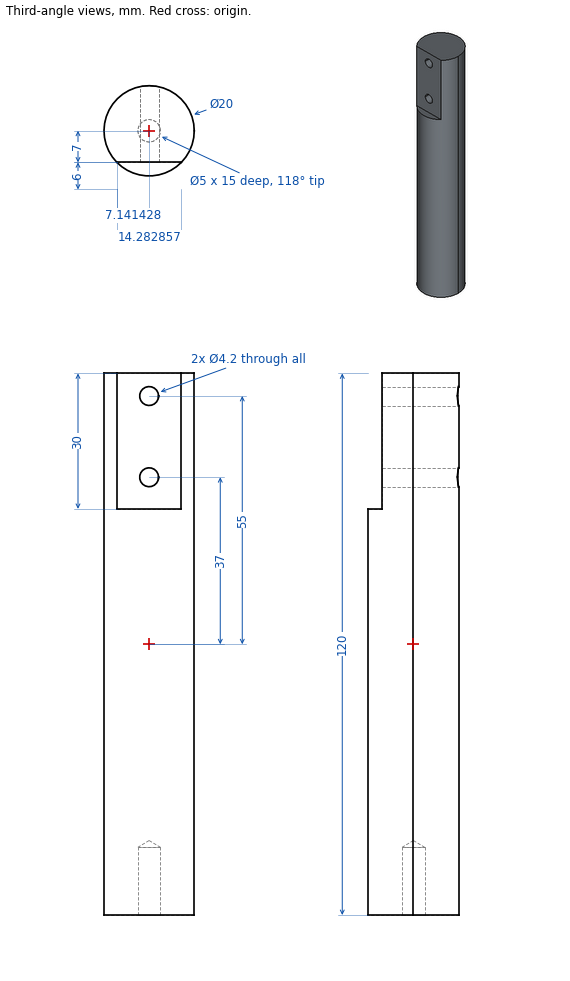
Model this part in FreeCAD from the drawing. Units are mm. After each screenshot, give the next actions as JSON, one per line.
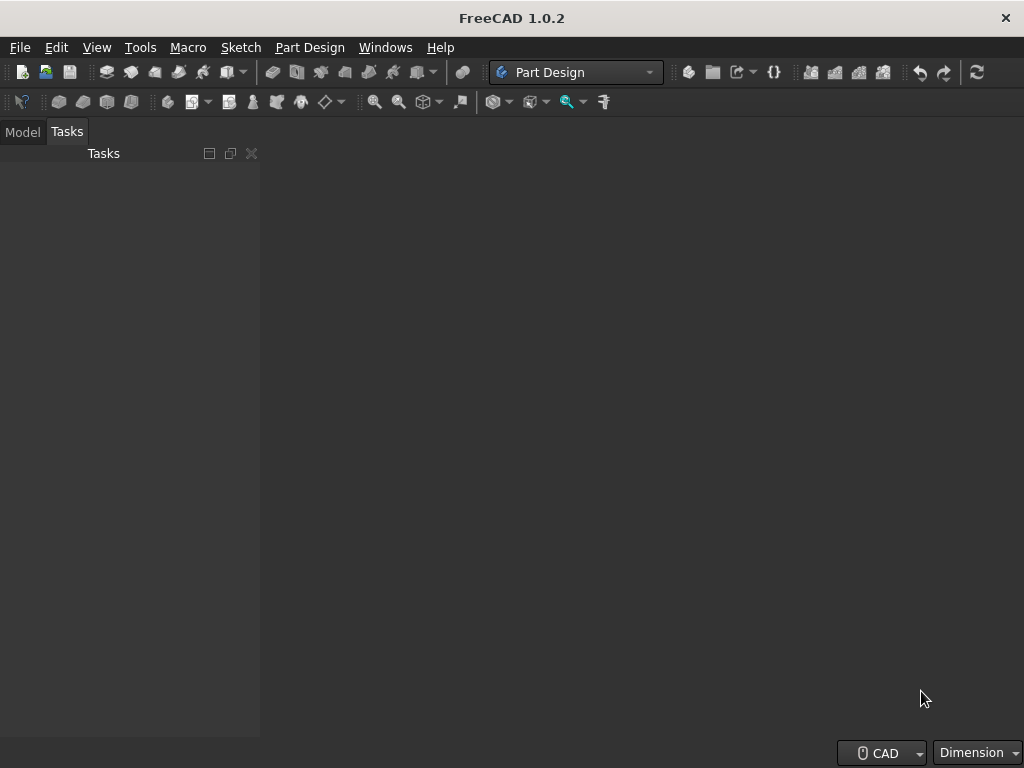
{"action": "left_click", "coordinate": [22, 72]}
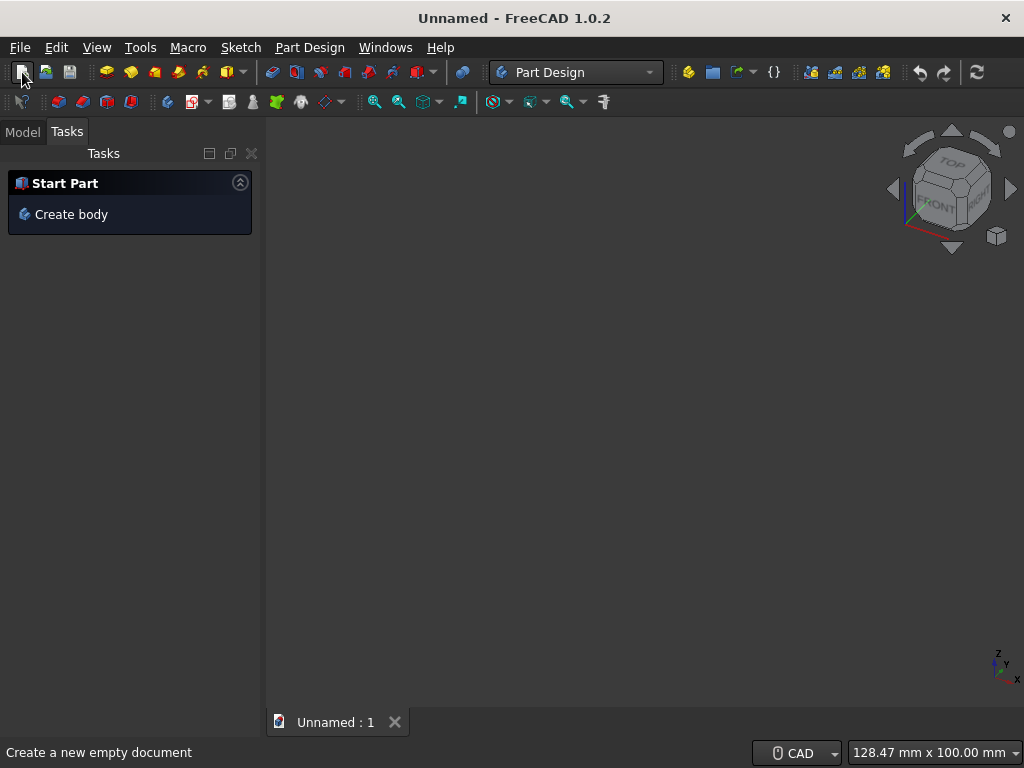
{"action": "left_click", "coordinate": [192, 102]}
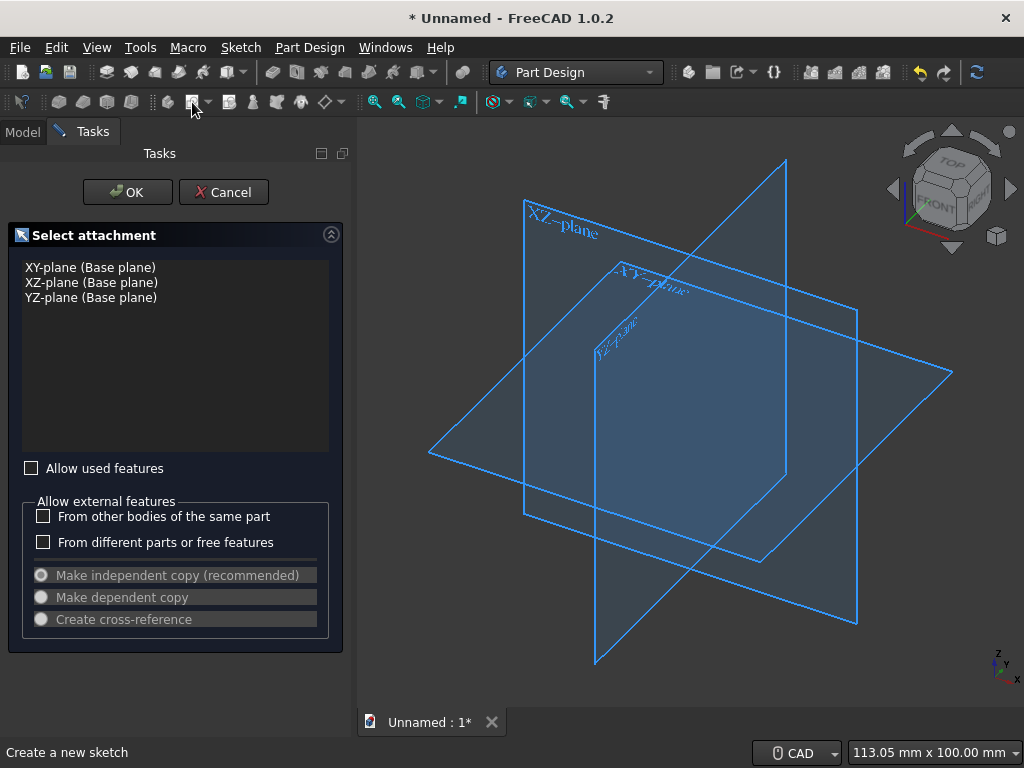
{"action": "left_click", "coordinate": [82, 268]}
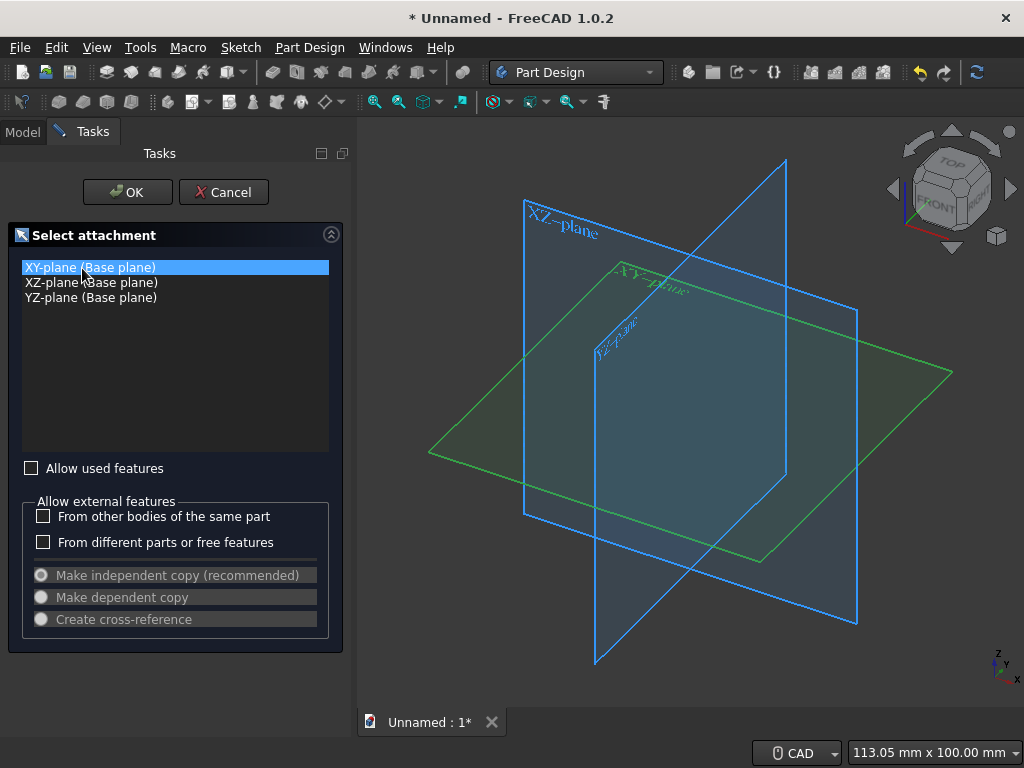
{"action": "left_click", "coordinate": [128, 192]}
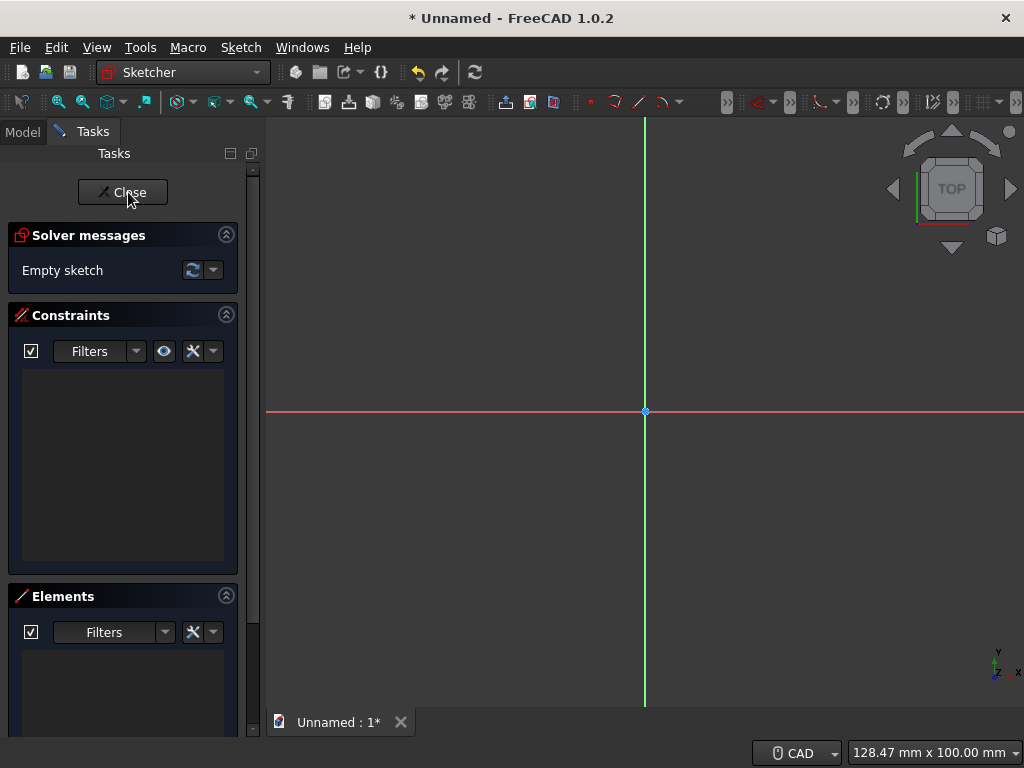
{"action": "scroll", "coordinate": [675, 412], "scroll_direction": "up", "scroll_amount": 6}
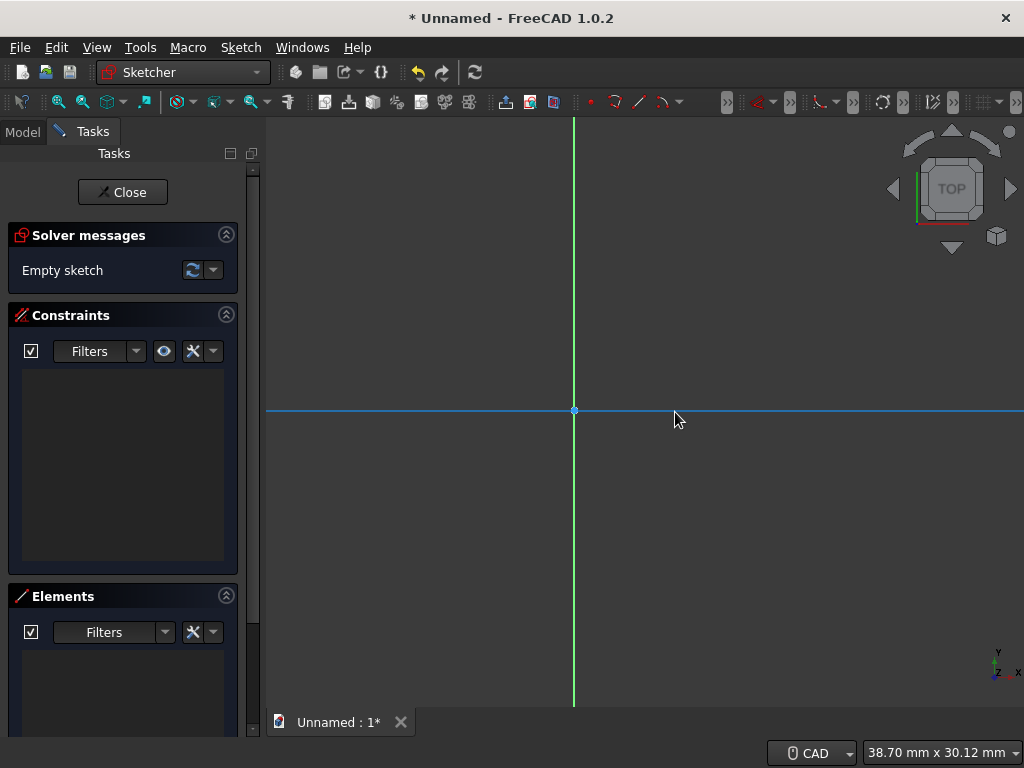
{"action": "key", "text": "g c"}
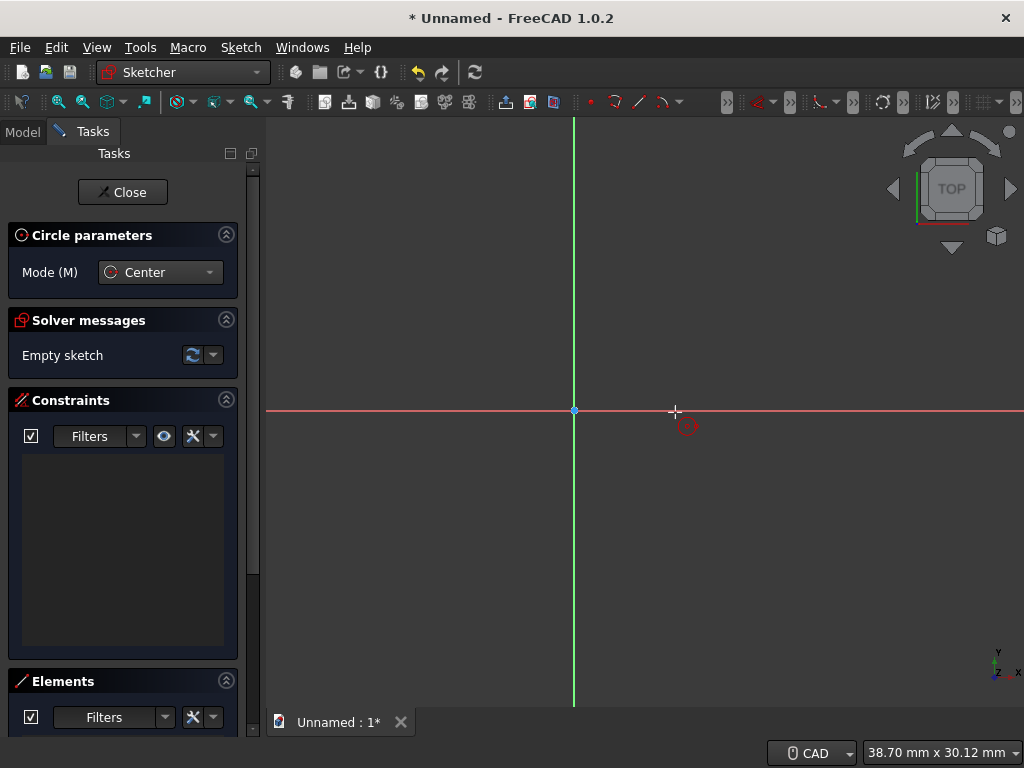
{"action": "left_click", "coordinate": [574, 411]}
{"action": "left_click", "coordinate": [713, 272]}
{"action": "key", "text": "Escape"}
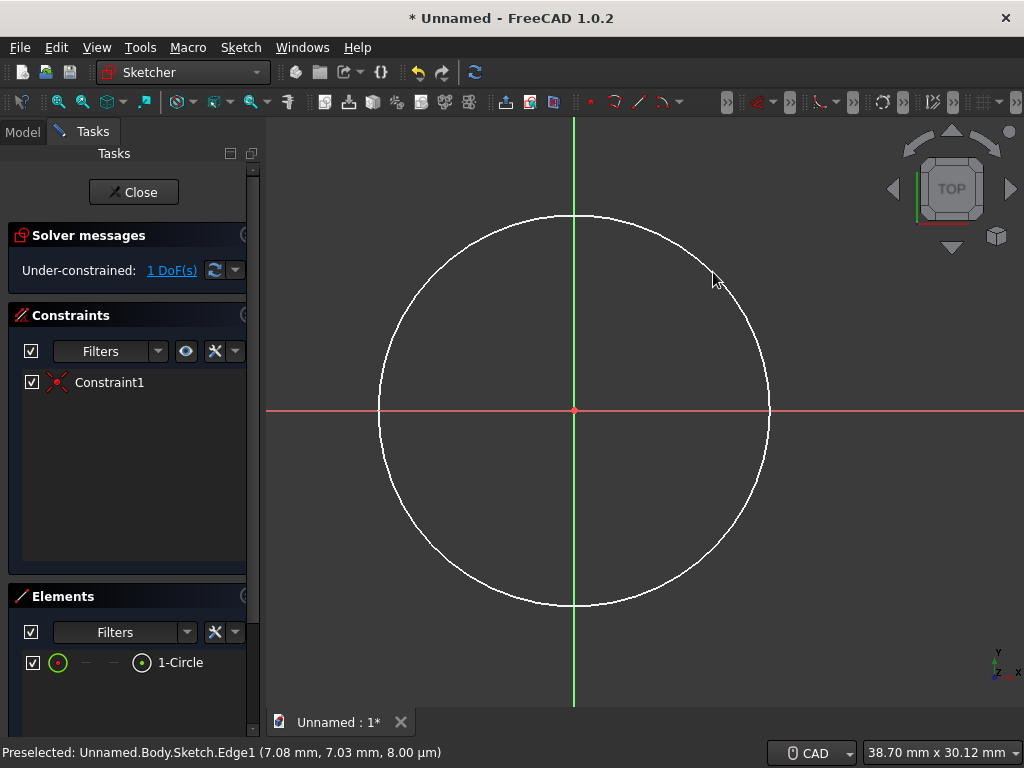
{"action": "left_click", "coordinate": [758, 102]}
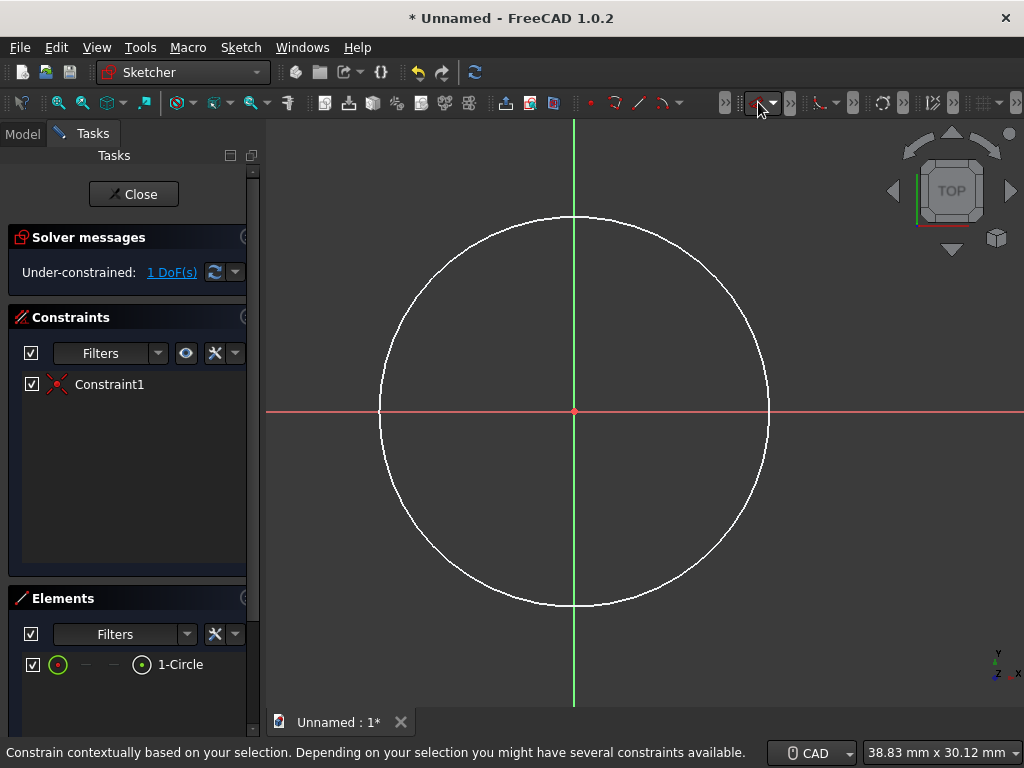
{"action": "left_click", "coordinate": [712, 274]}
{"action": "left_click", "coordinate": [735, 251]}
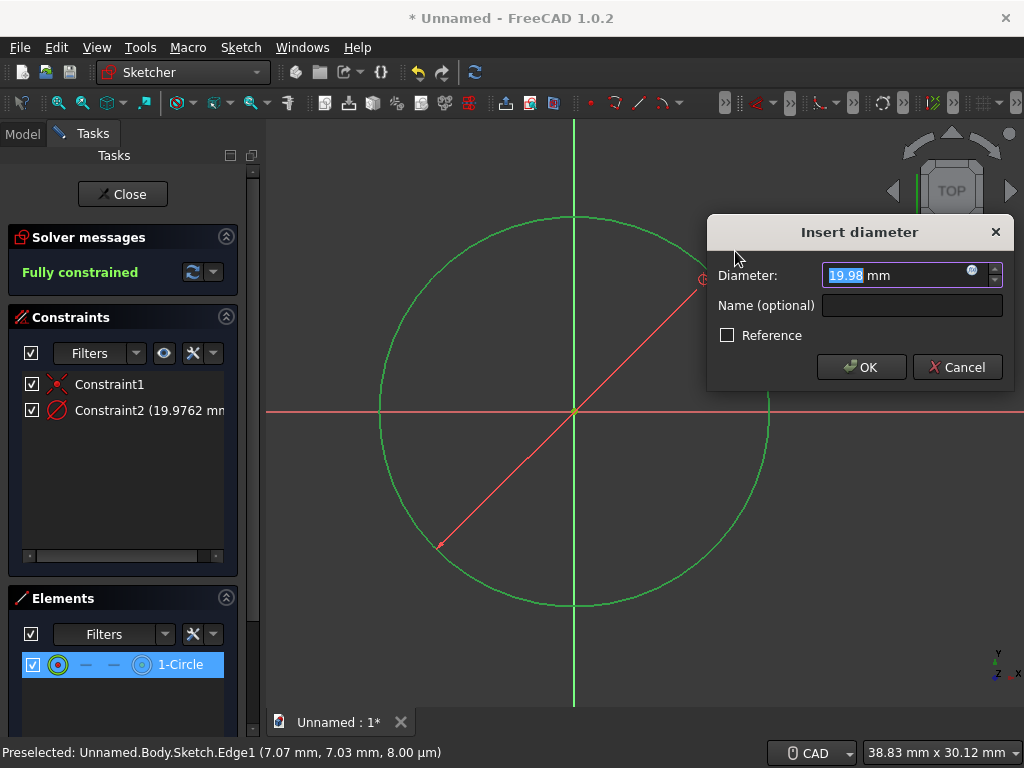
{"action": "type", "text": "20"}
{"action": "key", "text": "Return"}
{"action": "key", "text": "Escape"}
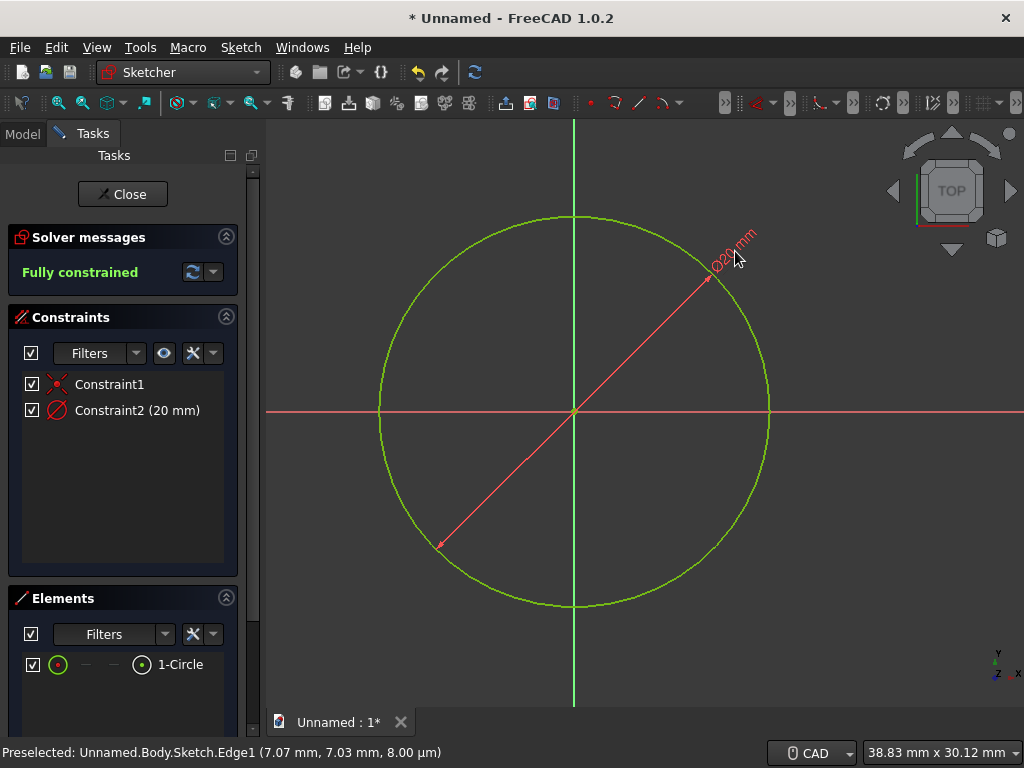
{"action": "left_click", "coordinate": [123, 194]}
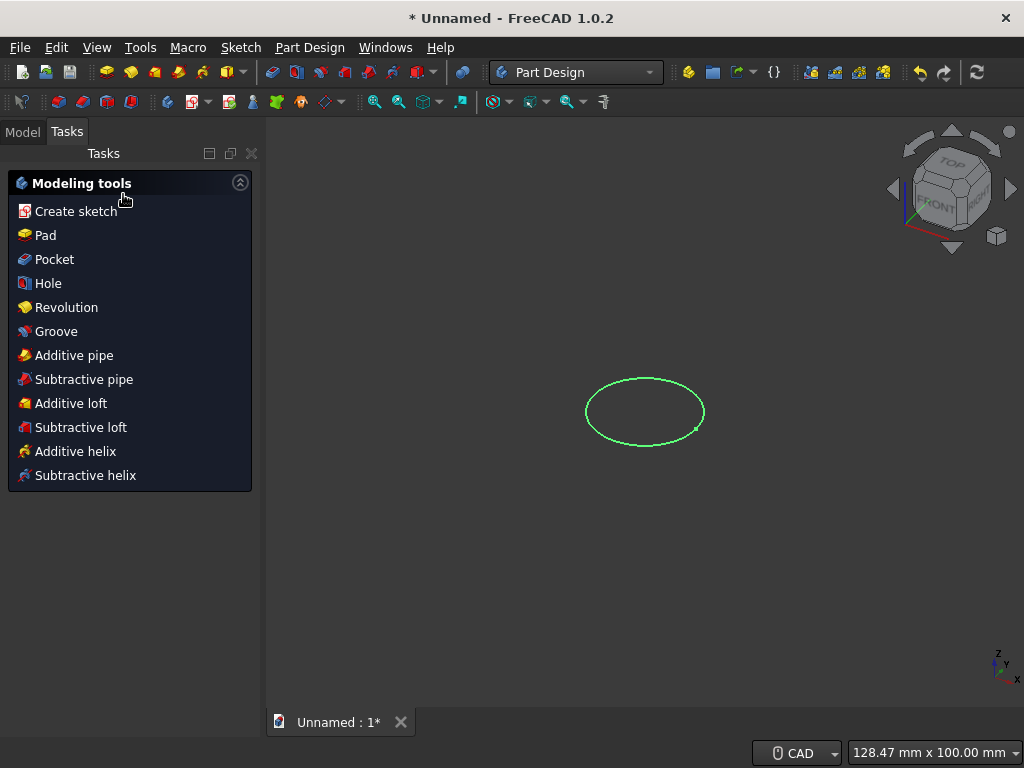
{"action": "left_click", "coordinate": [108, 72]}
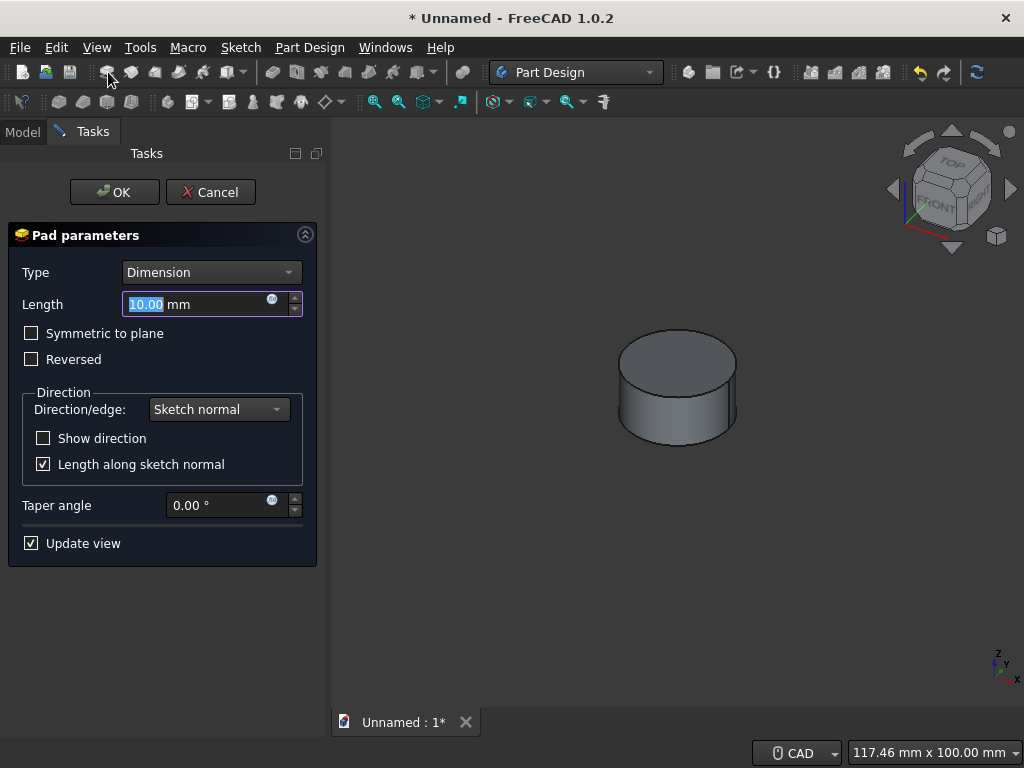
{"action": "type", "text": "120"}
{"action": "key", "text": "Tab"}